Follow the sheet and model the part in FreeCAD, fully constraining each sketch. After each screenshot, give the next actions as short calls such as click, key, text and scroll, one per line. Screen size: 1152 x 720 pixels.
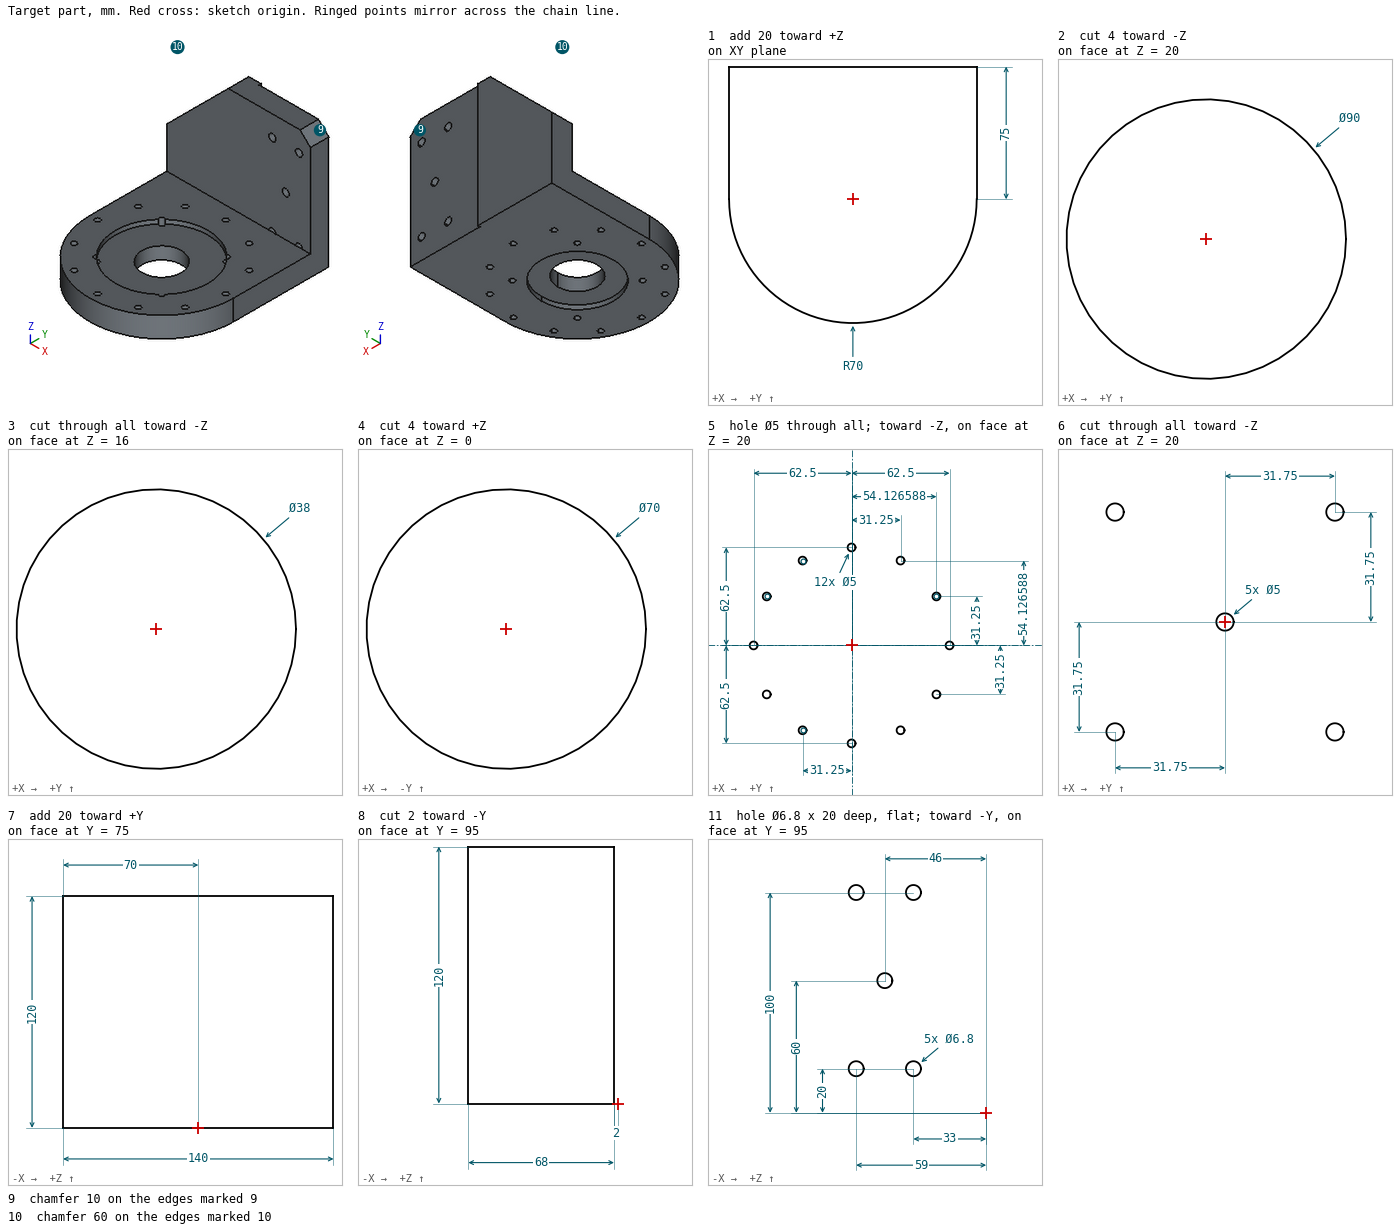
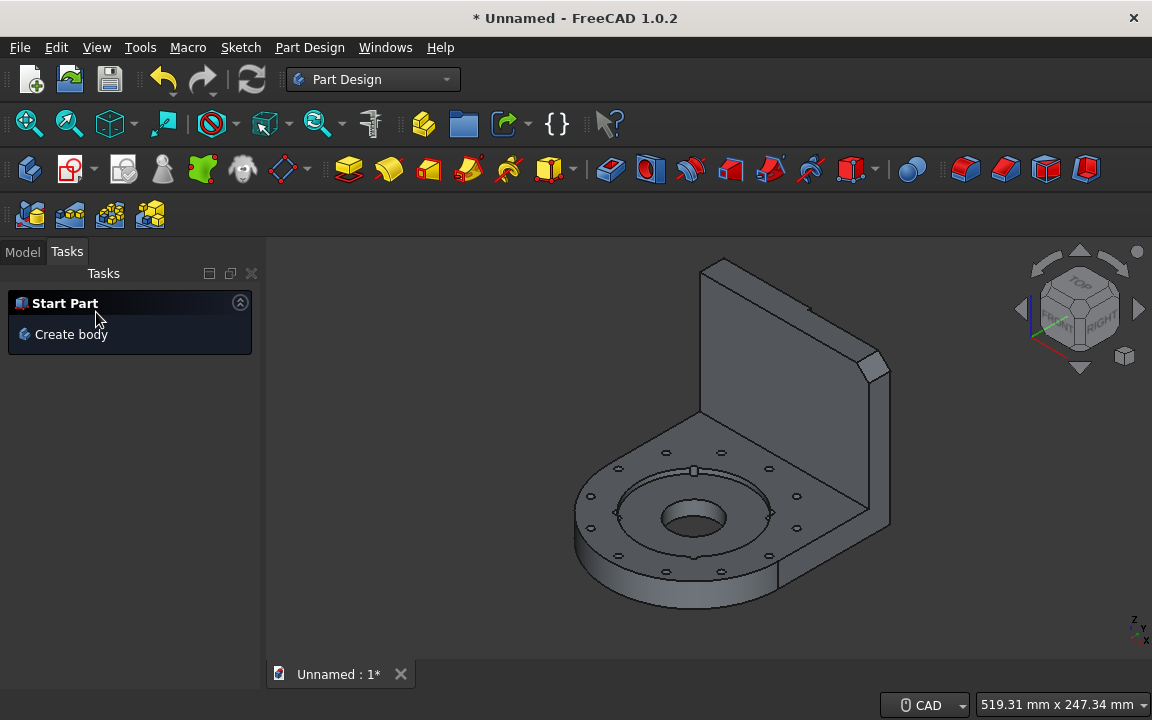
key(2)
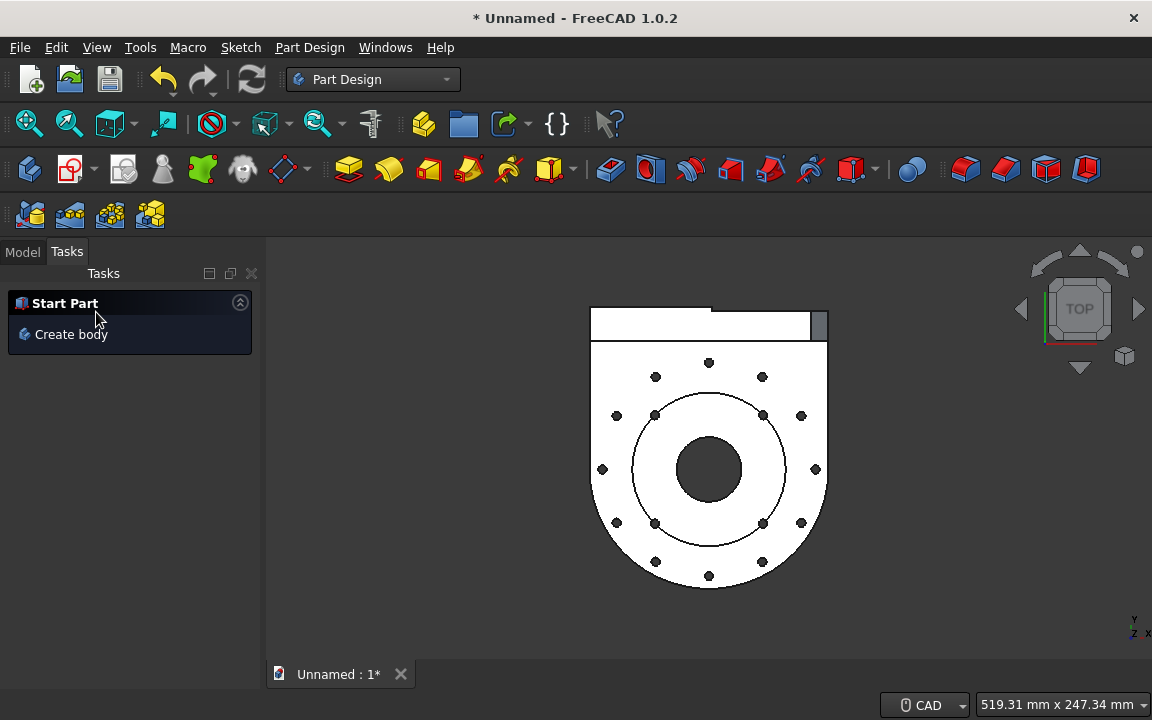
click(590, 323)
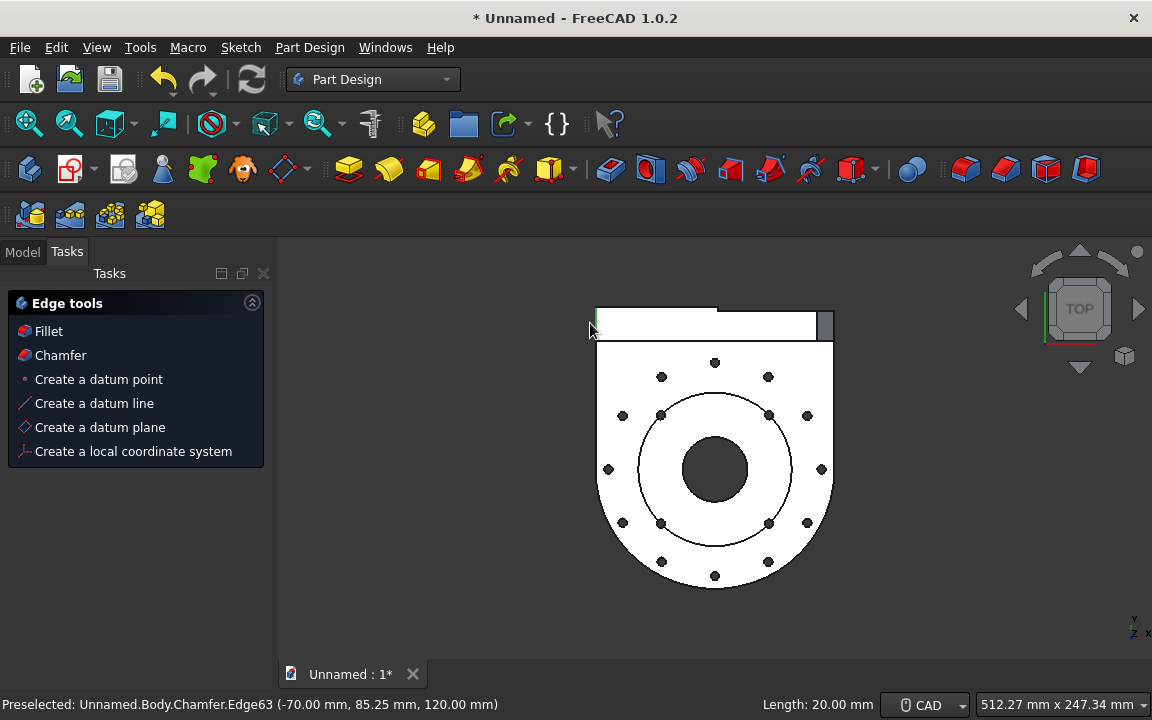
click(1006, 170)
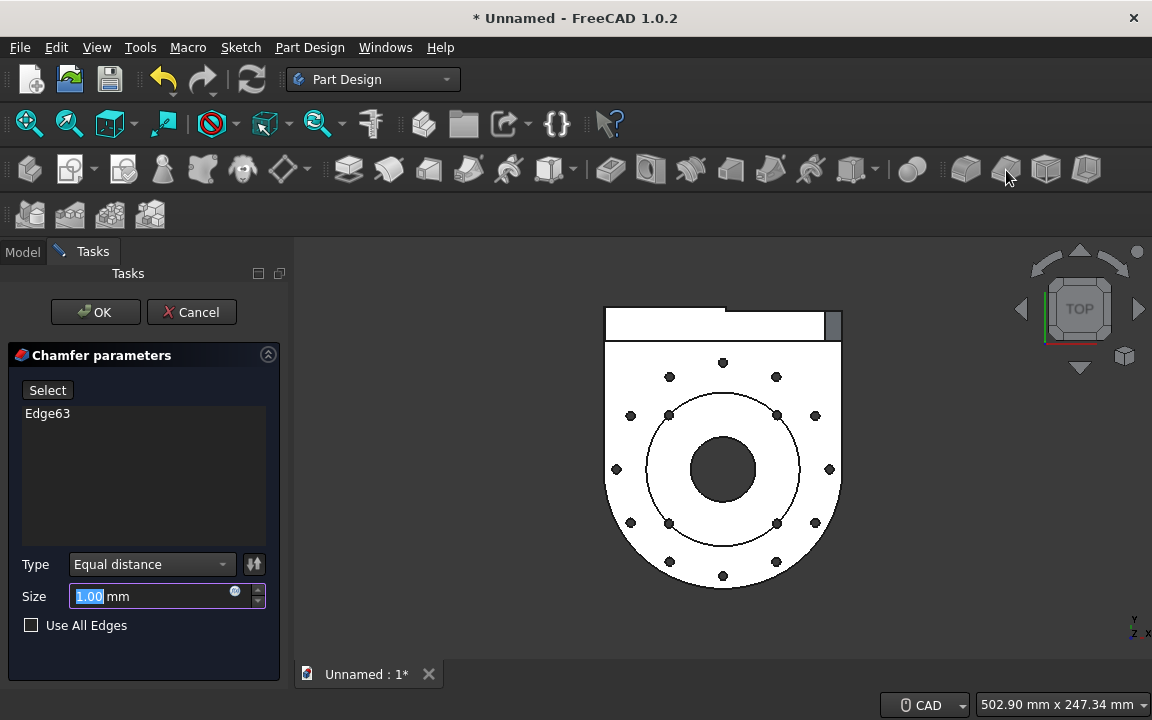
text(60)
key(Tab)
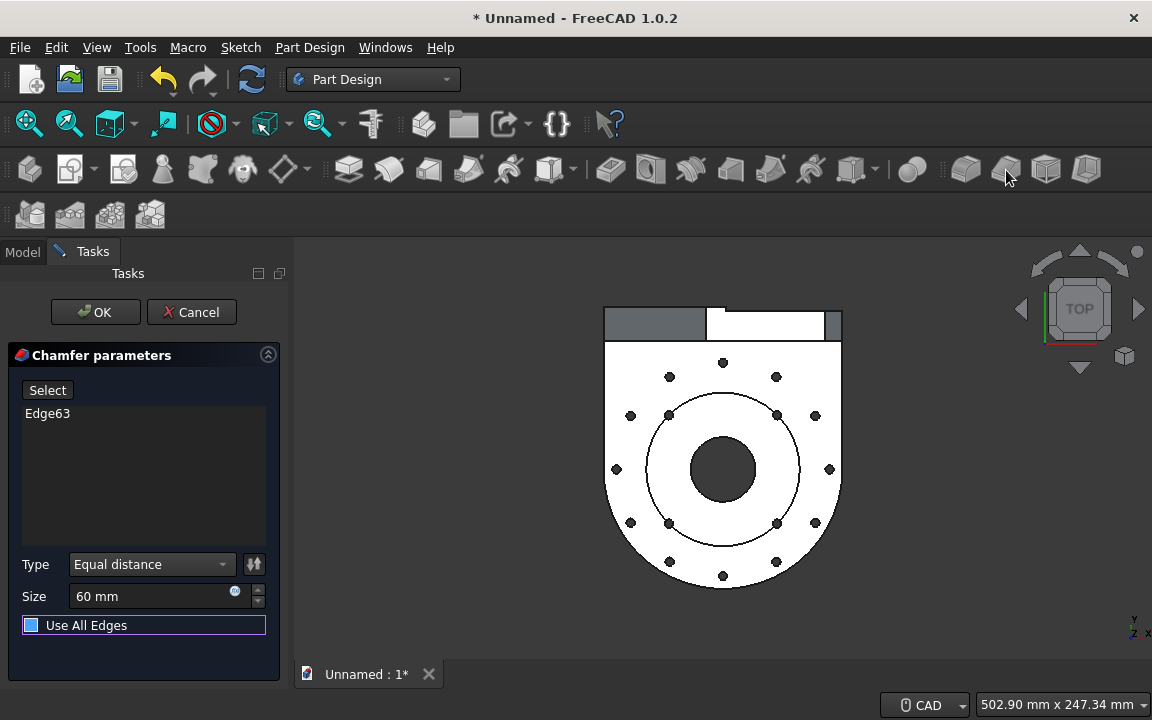
click(96, 312)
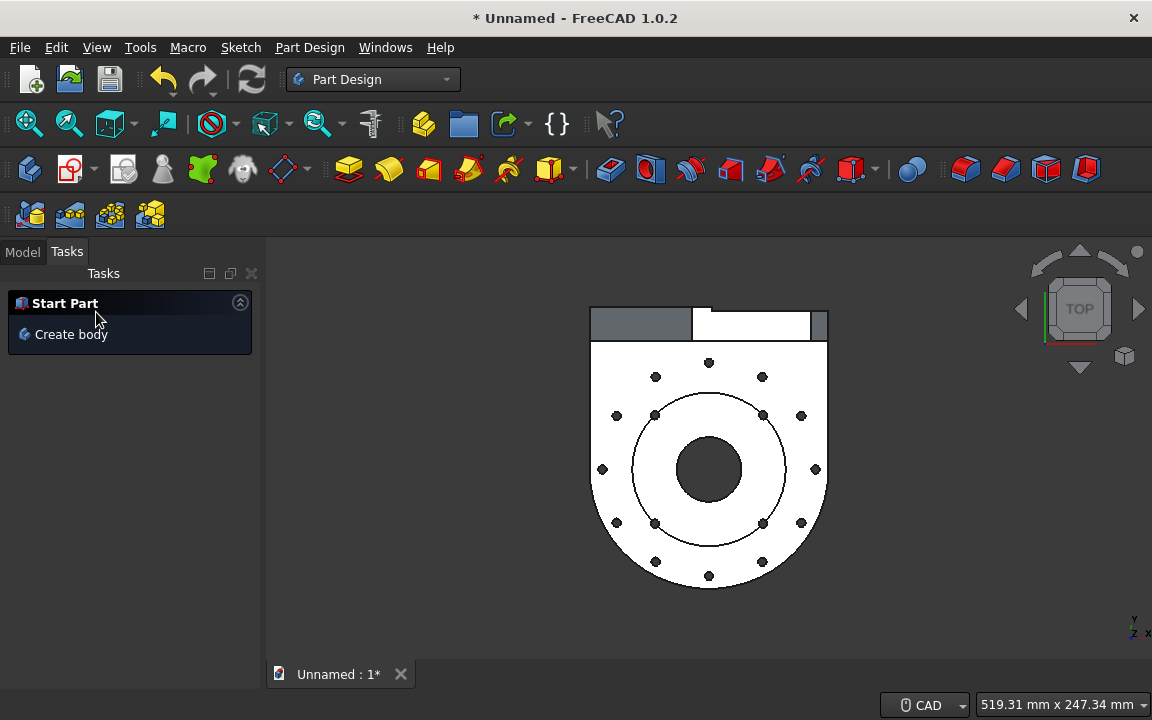
key(4)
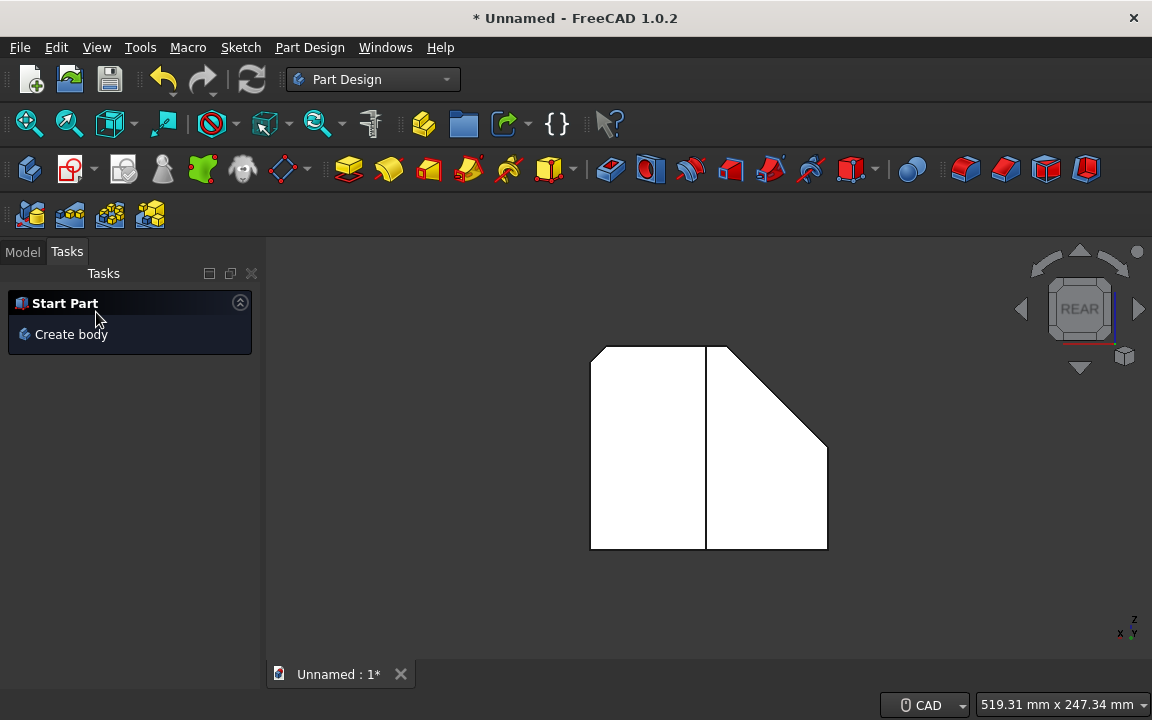
click(767, 476)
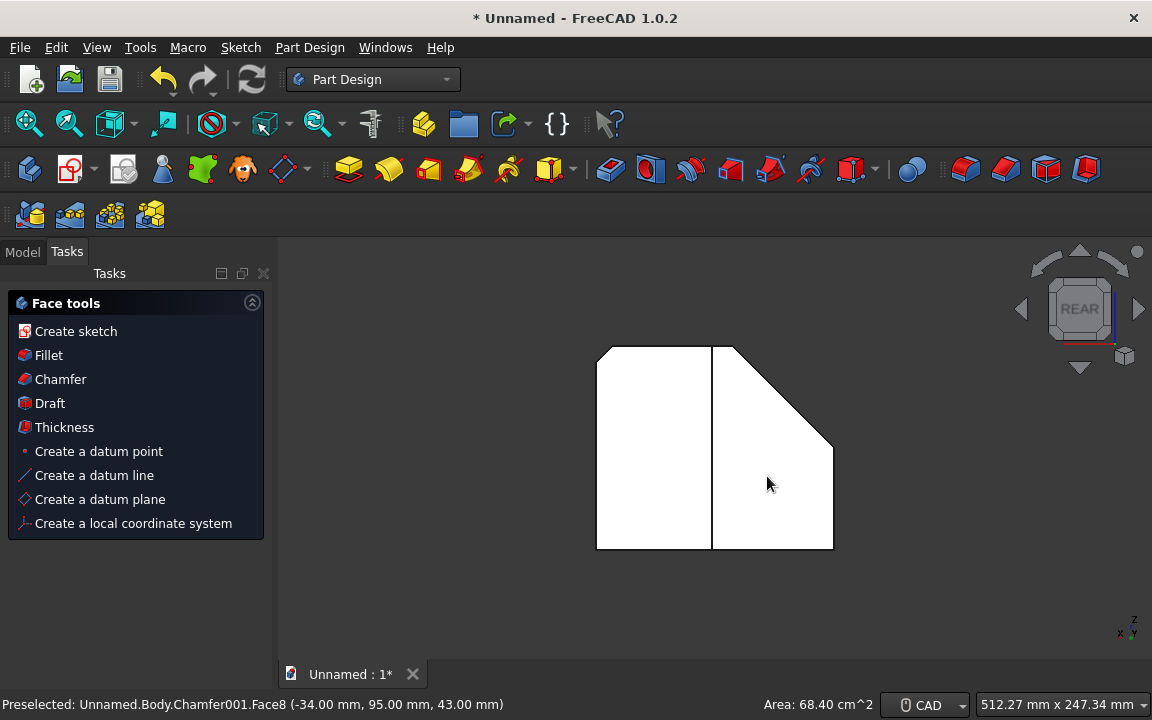
click(70, 170)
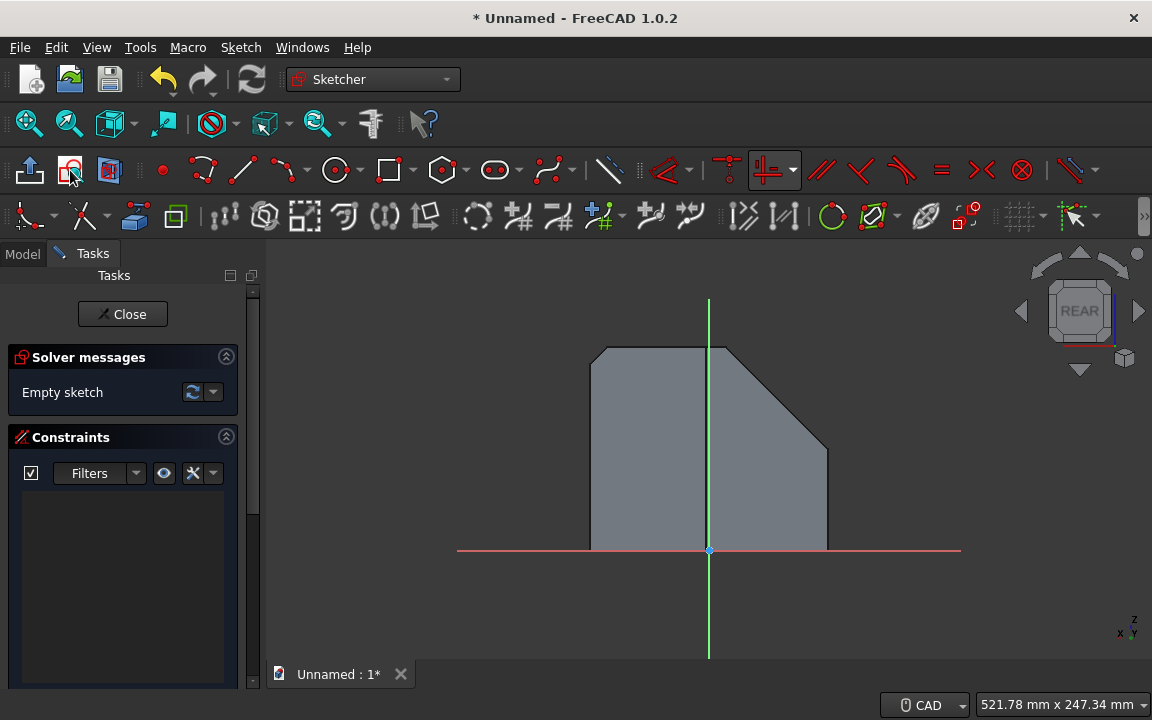
scroll(688, 492, up, 2)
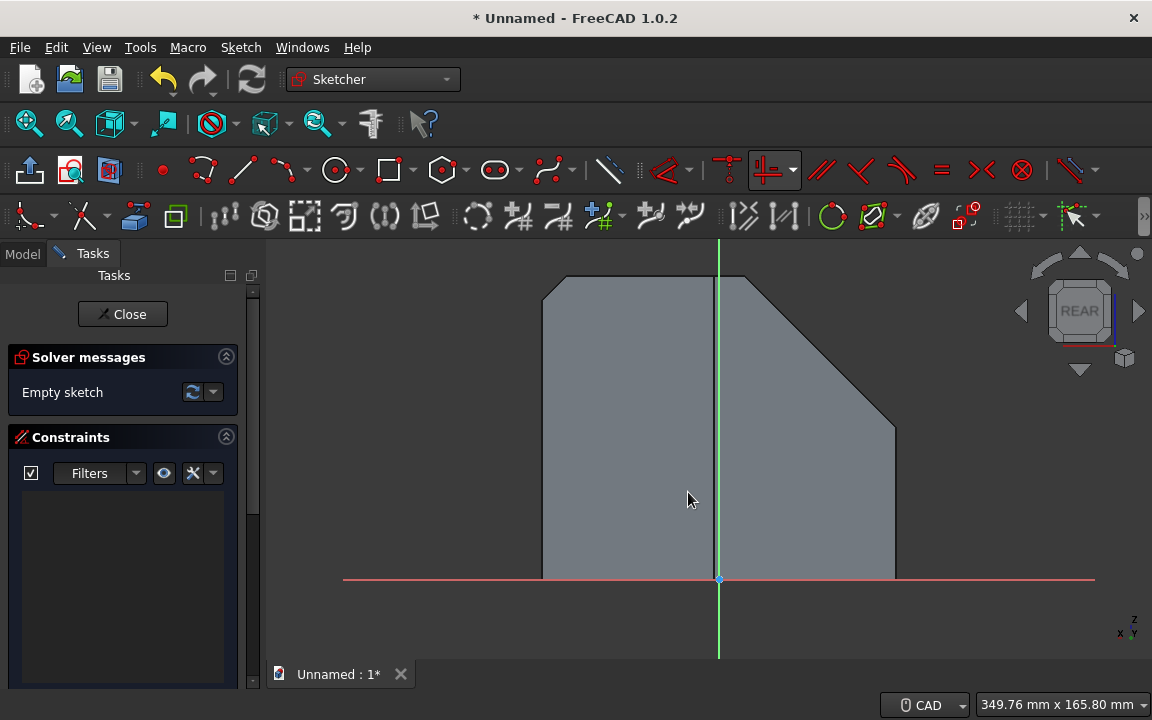
click(336, 170)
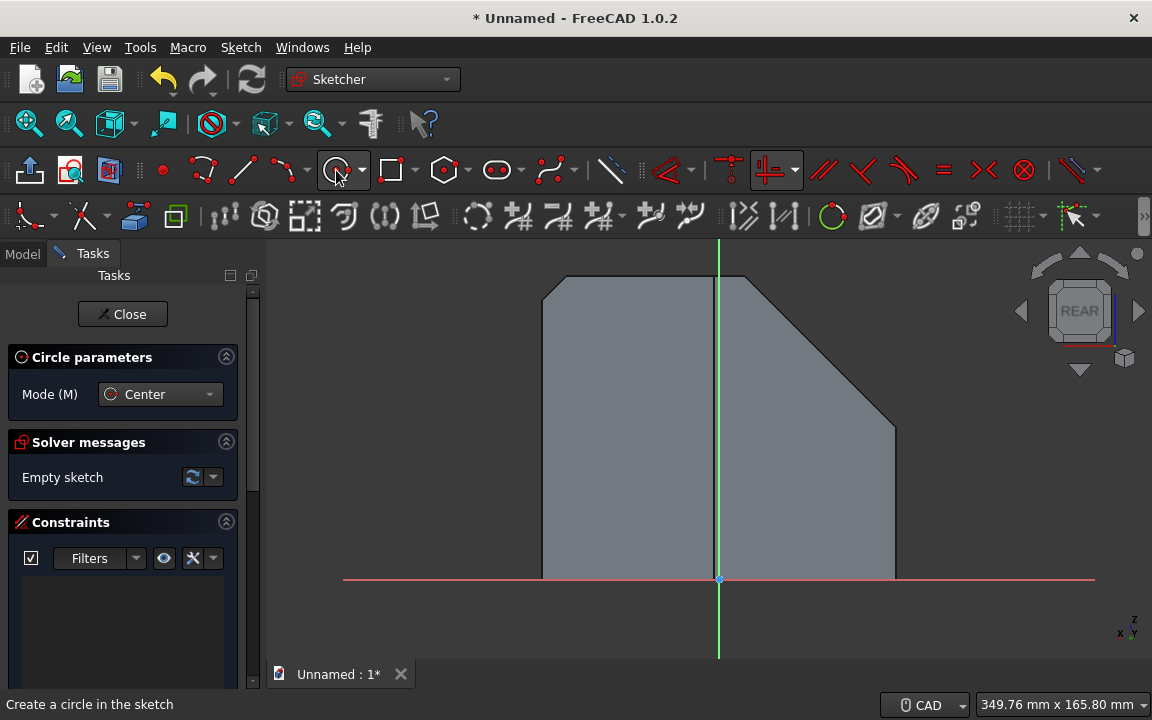
scroll(635, 529, up, 5)